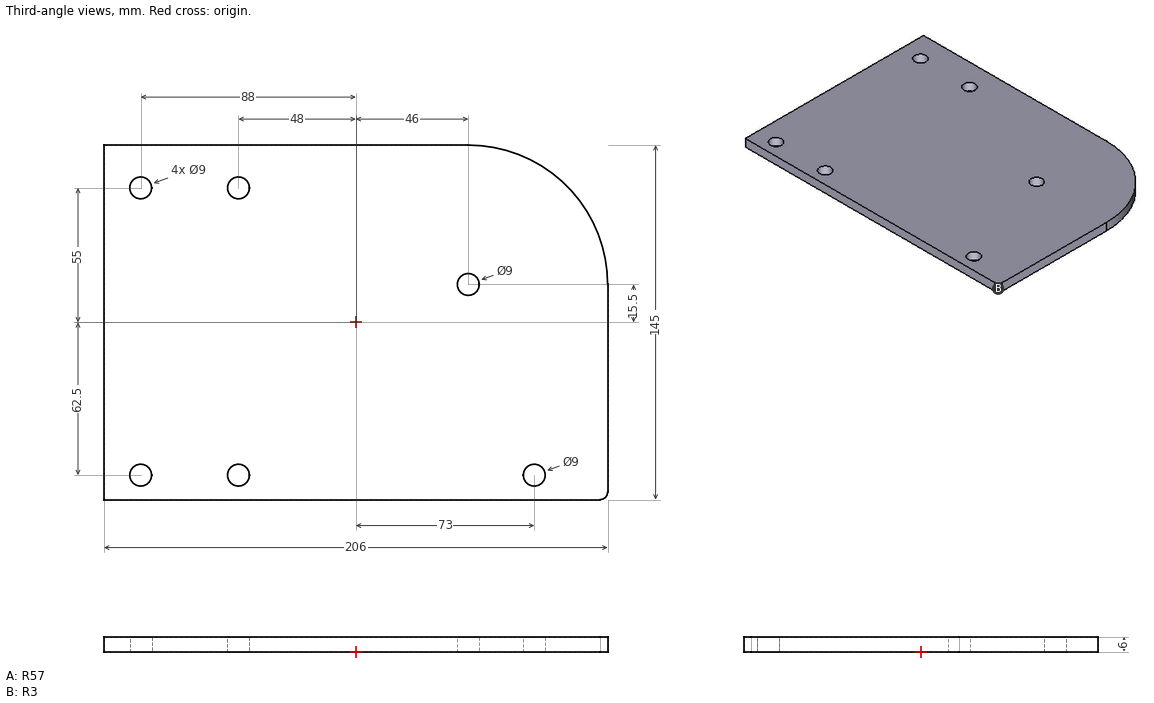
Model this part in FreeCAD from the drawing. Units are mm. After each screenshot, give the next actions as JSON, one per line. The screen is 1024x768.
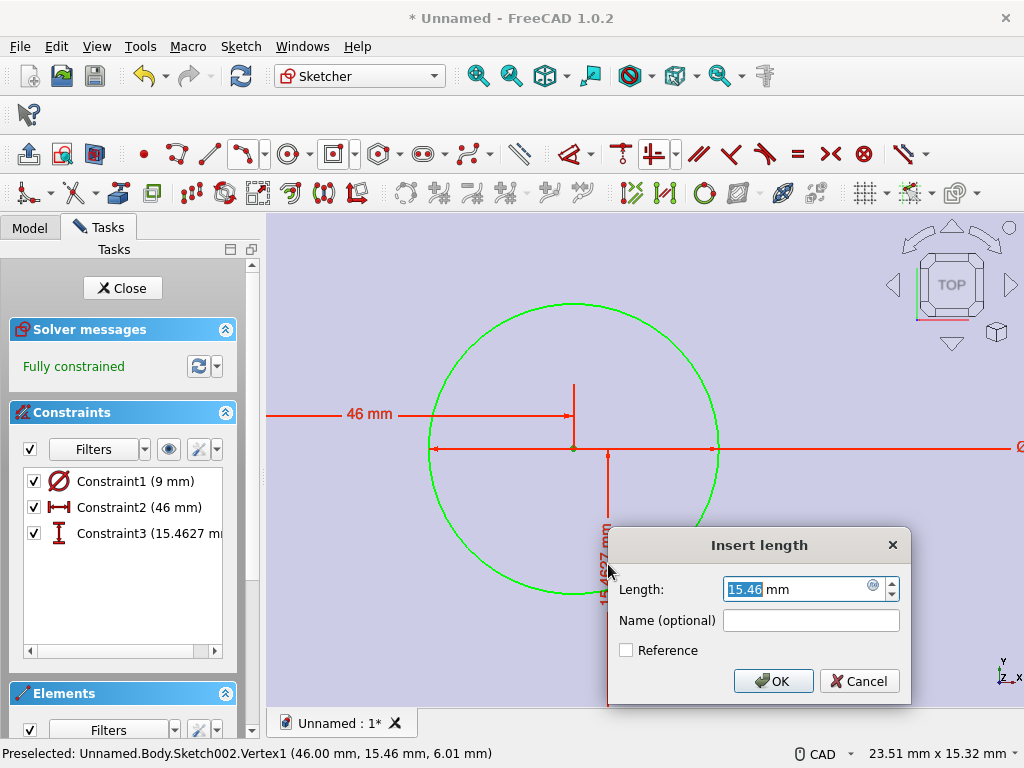
{"action": "type", "text": "15.5"}
{"action": "key", "text": "Return"}
{"action": "key", "text": "Escape"}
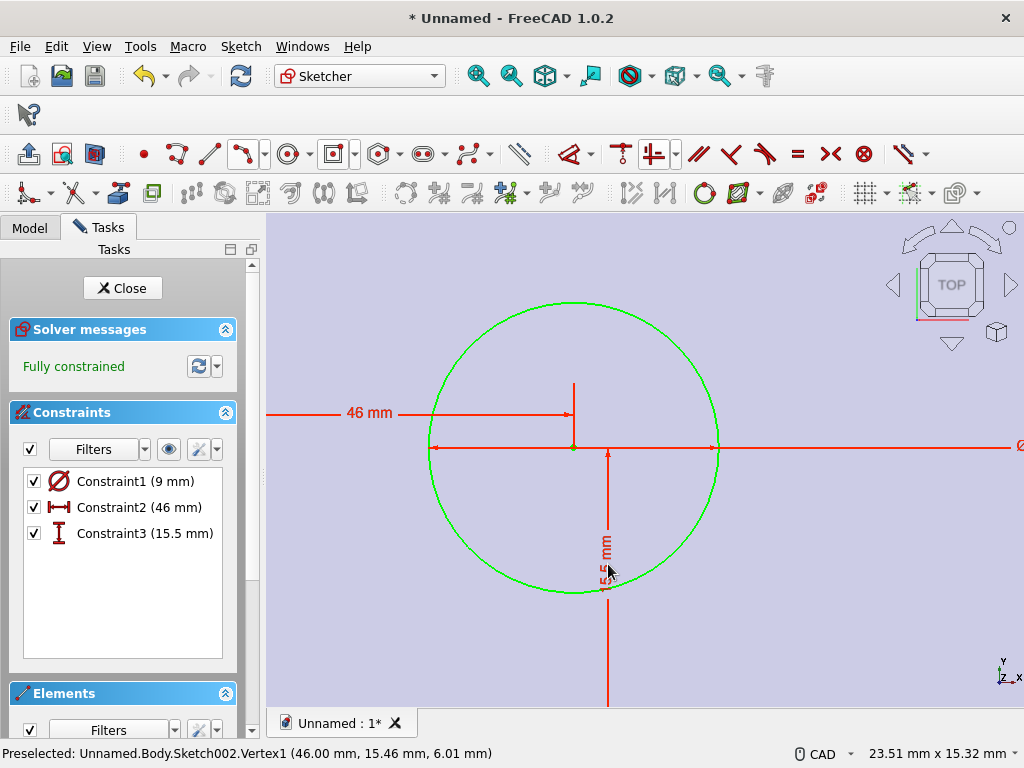
{"action": "left_click", "coordinate": [123, 288]}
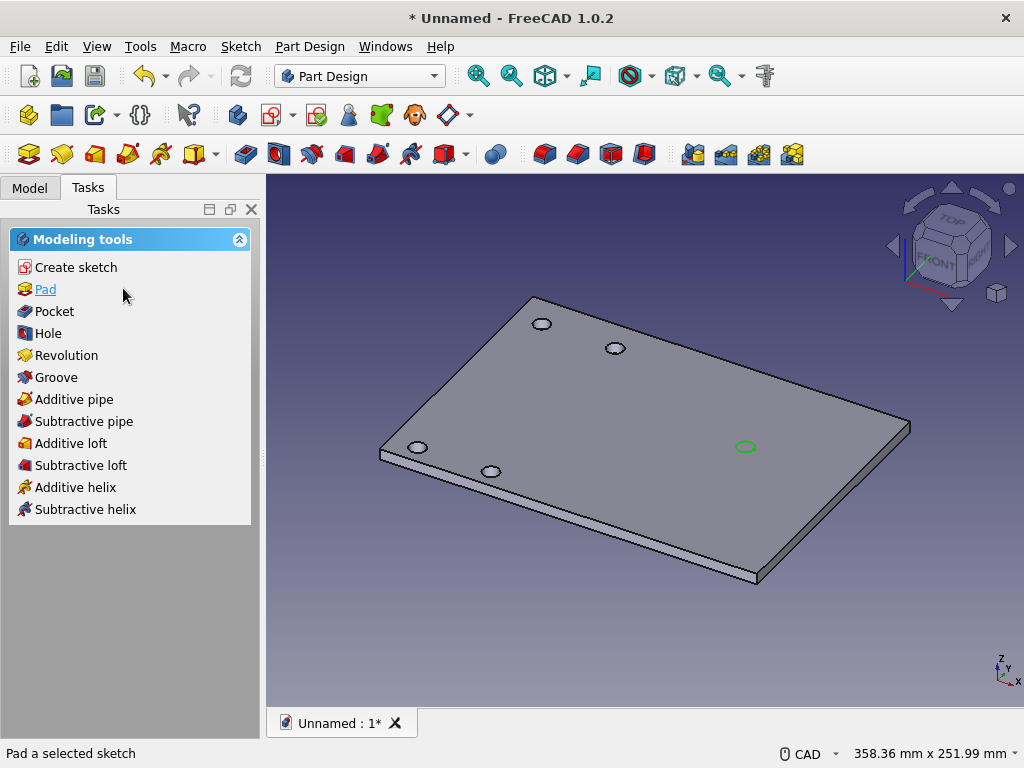
{"action": "left_click", "coordinate": [246, 154]}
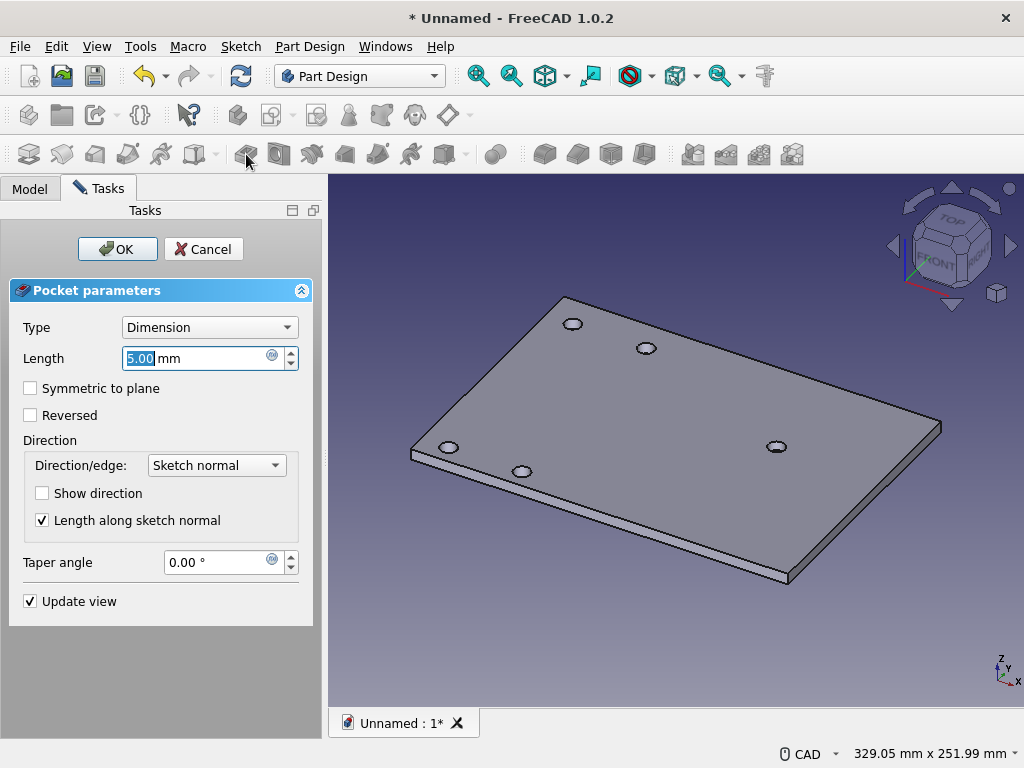
{"action": "left_click", "coordinate": [210, 328]}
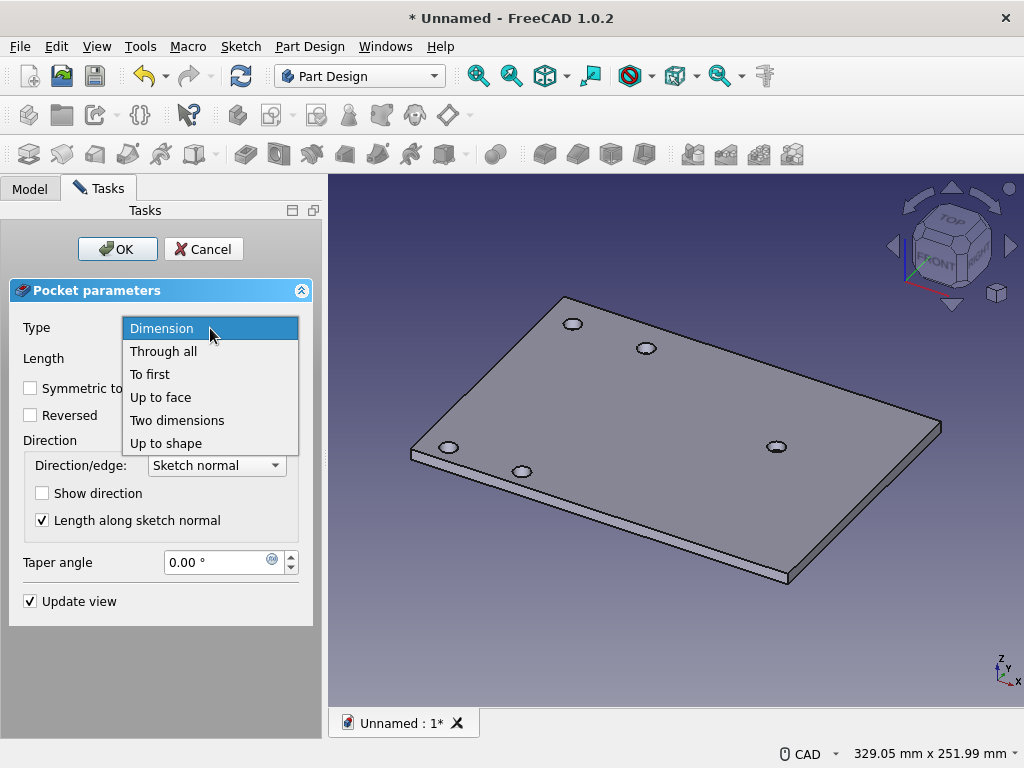
{"action": "left_click", "coordinate": [208, 352]}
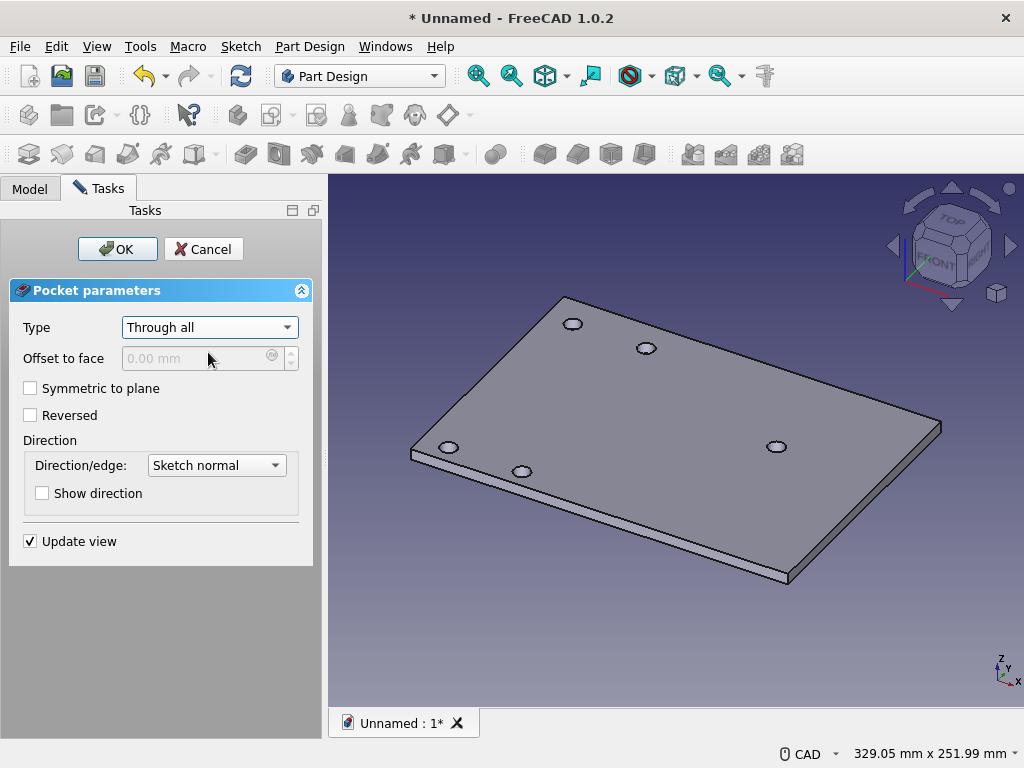
{"action": "left_click", "coordinate": [118, 249]}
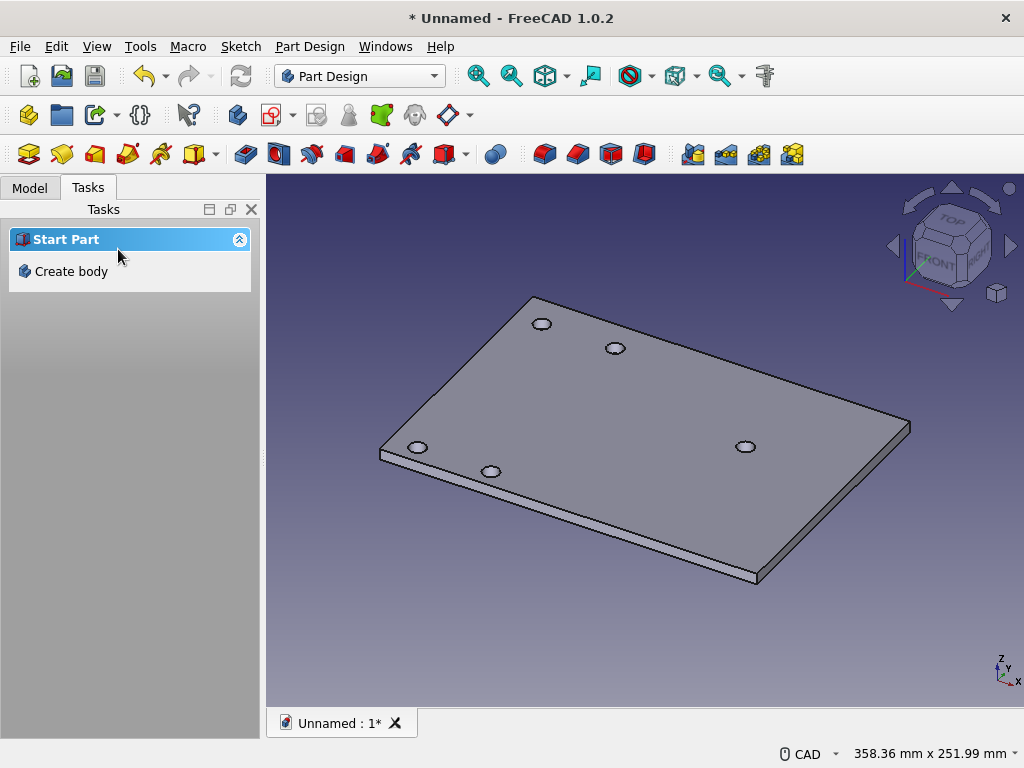
{"action": "key", "text": "0"}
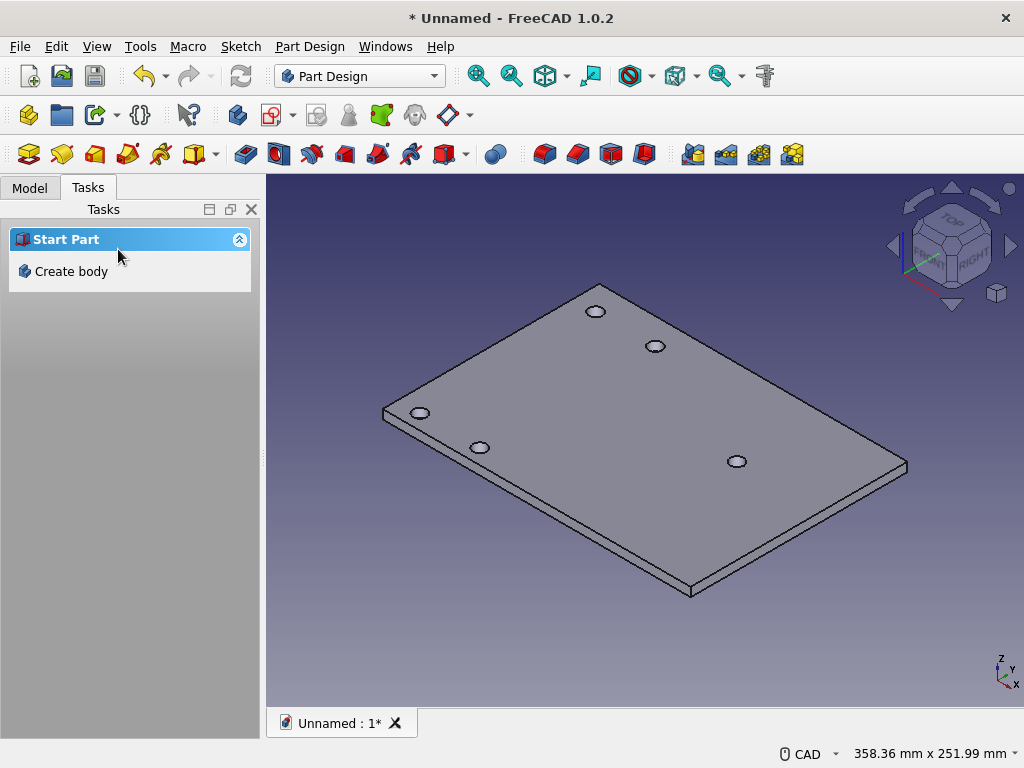
{"action": "key", "text": "2"}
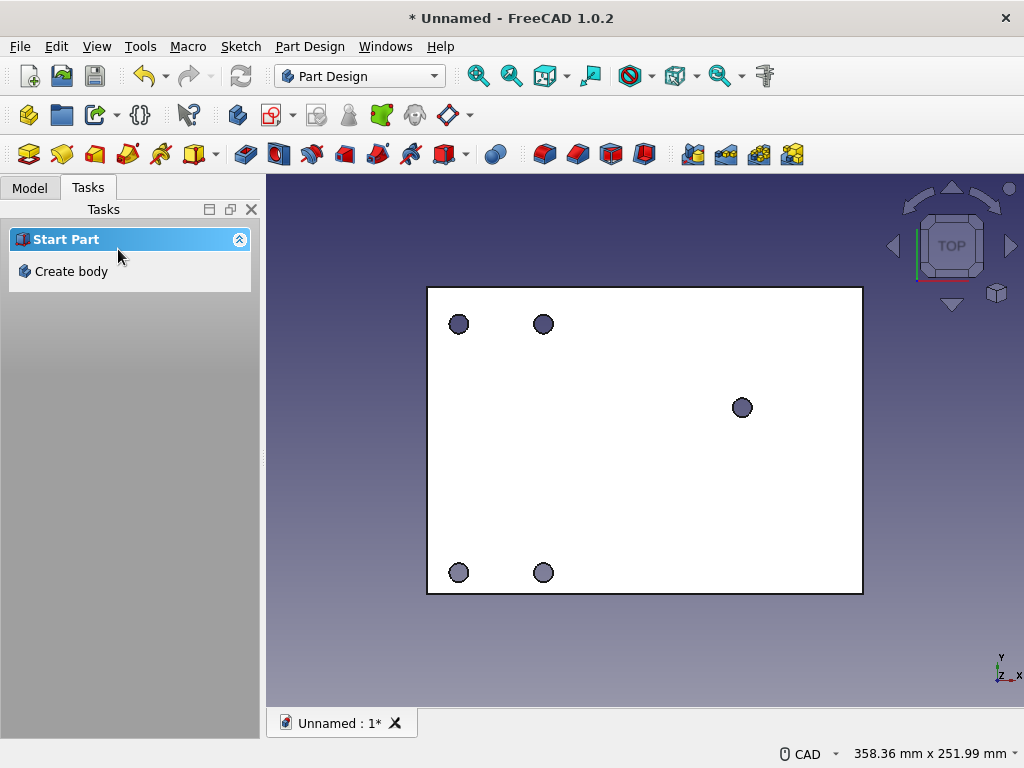
{"action": "key", "text": "1"}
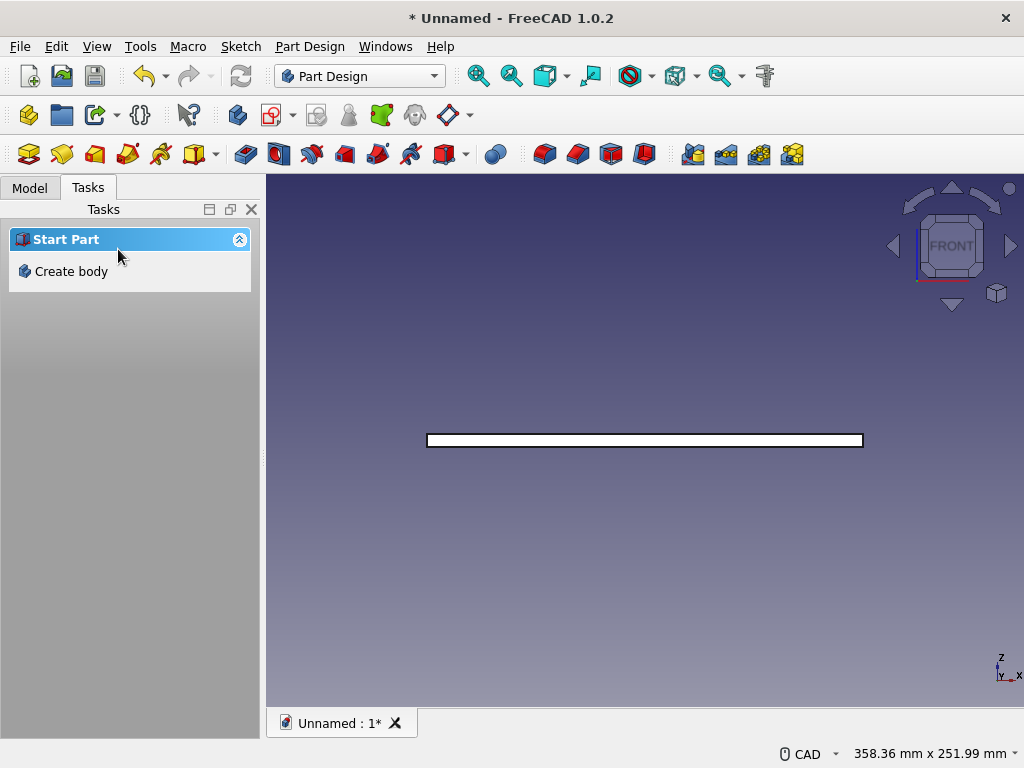
{"action": "key", "text": "3"}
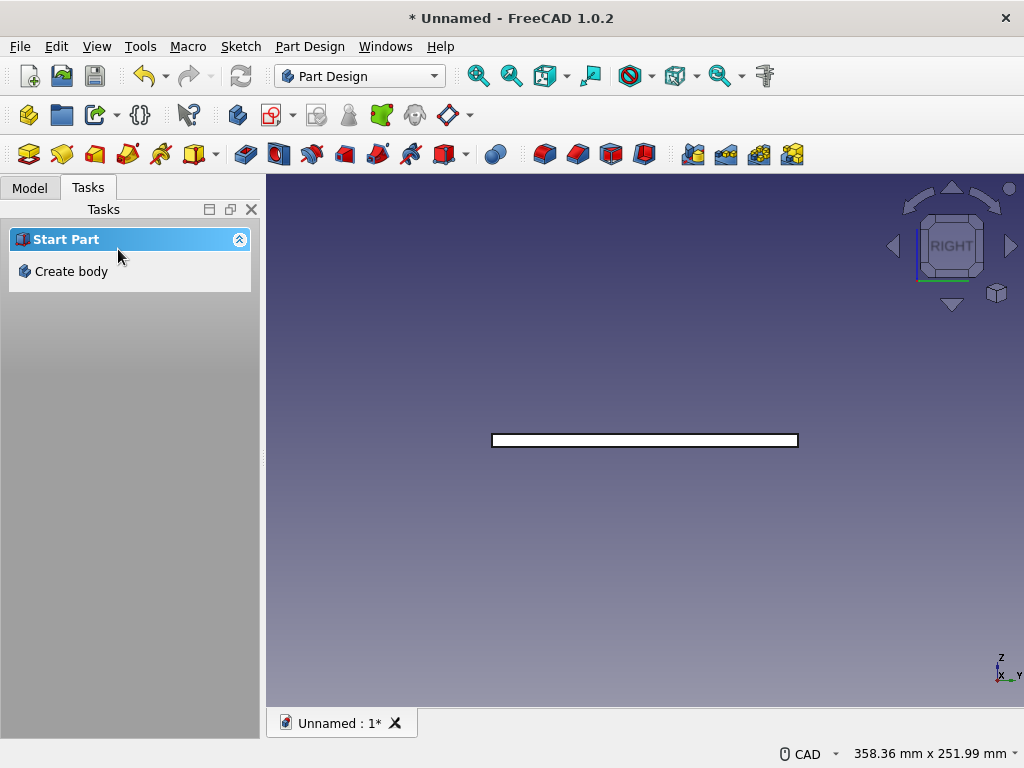
{"action": "left_click", "coordinate": [479, 76]}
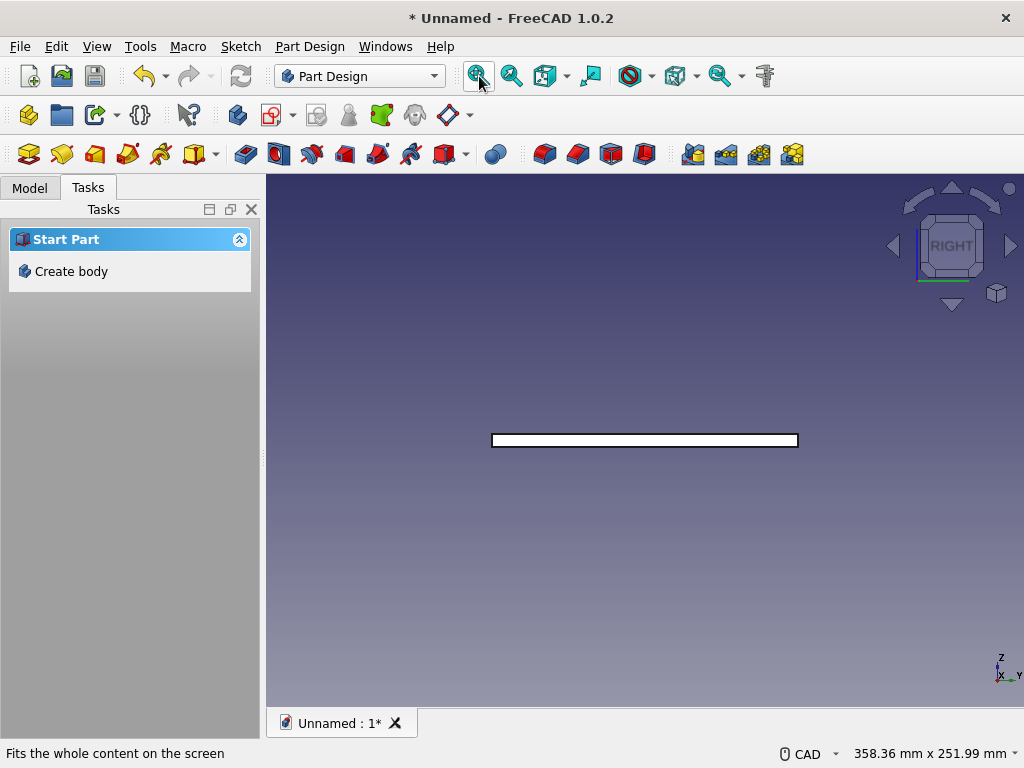
{"action": "scroll", "coordinate": [798, 439], "scroll_direction": "up", "scroll_amount": 6}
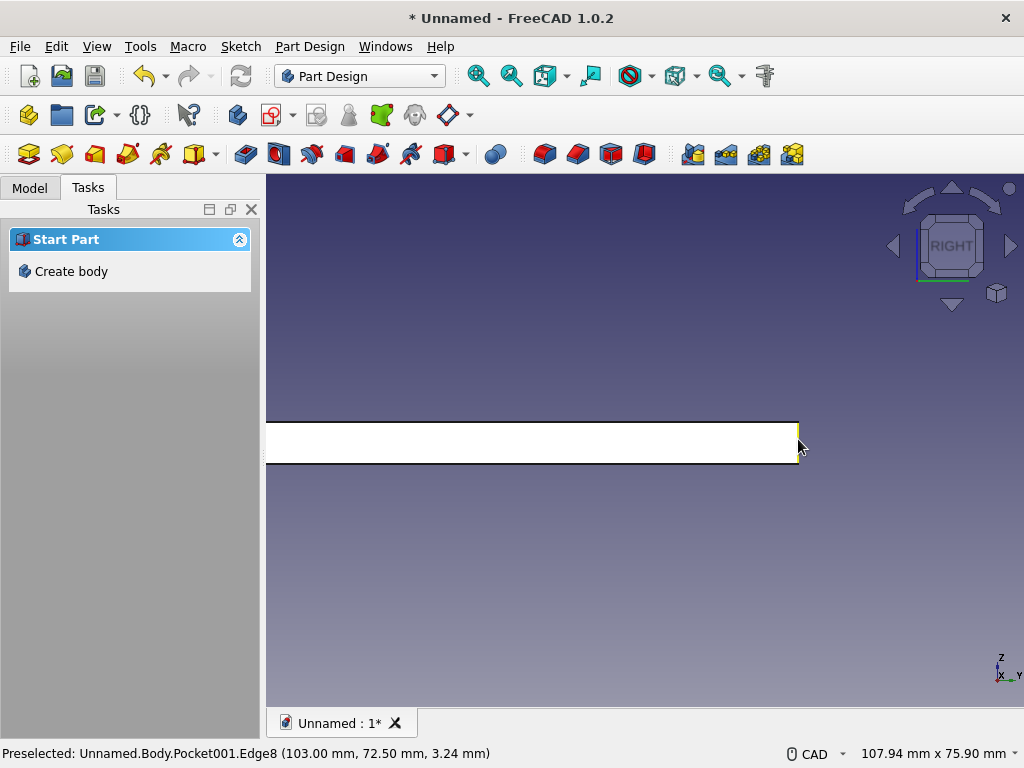
{"action": "left_click", "coordinate": [798, 442]}